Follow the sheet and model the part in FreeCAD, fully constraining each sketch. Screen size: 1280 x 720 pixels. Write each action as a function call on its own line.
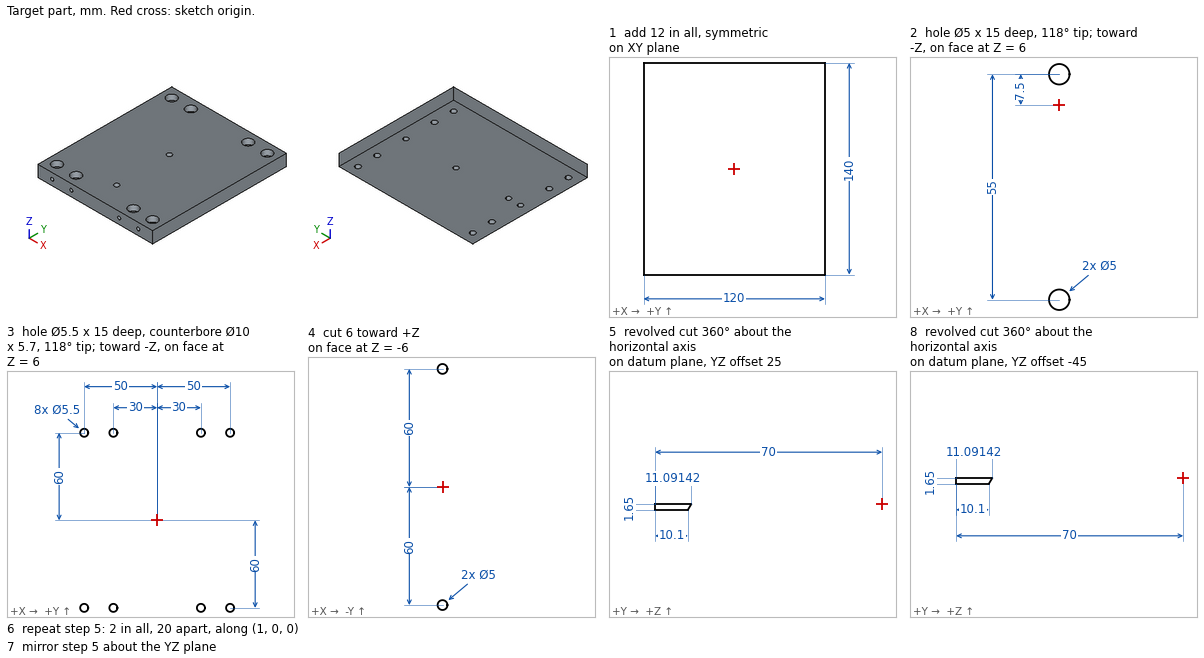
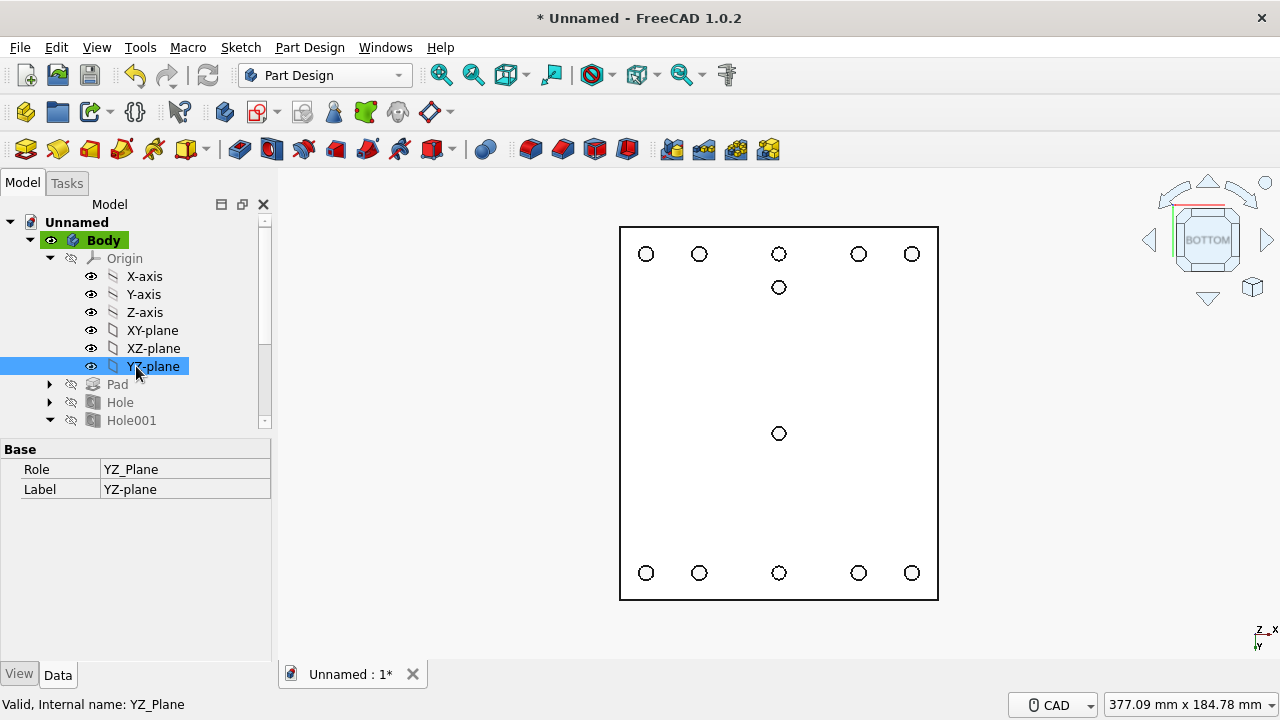
click(430, 112)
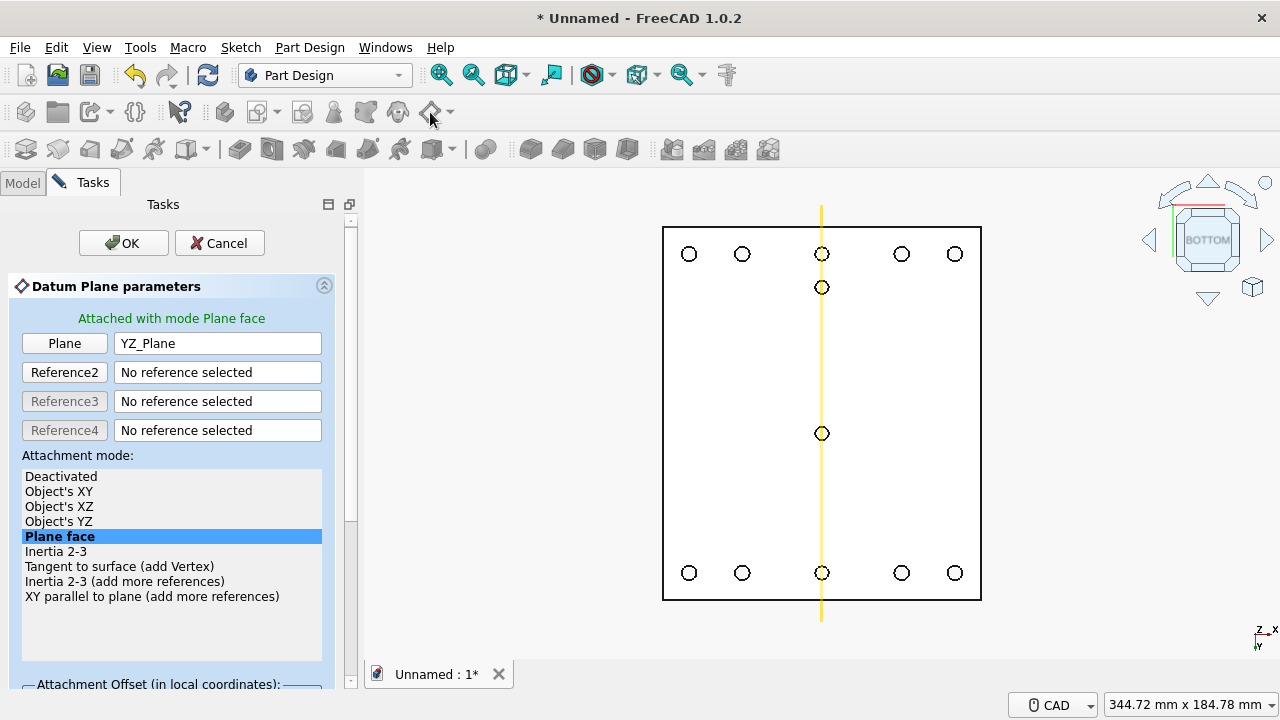
scroll(351, 451, down, 3)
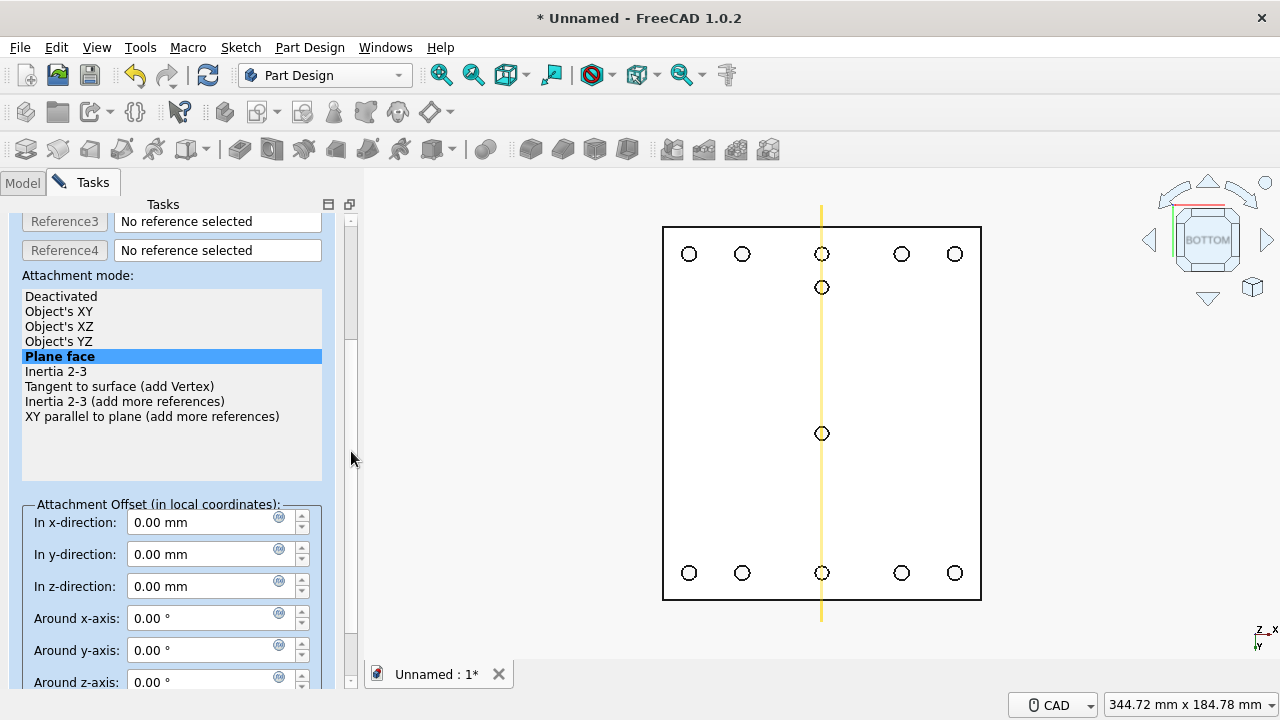
triple_click(210, 586)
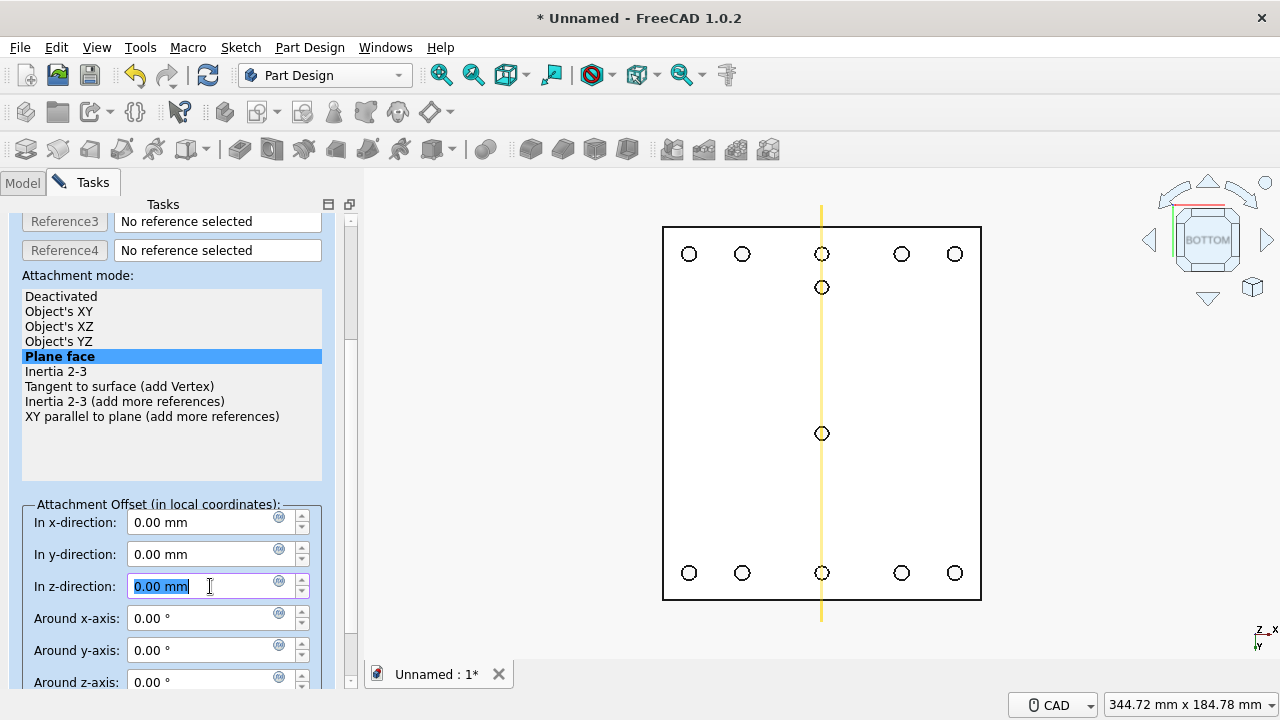
text(-45)
key(Tab)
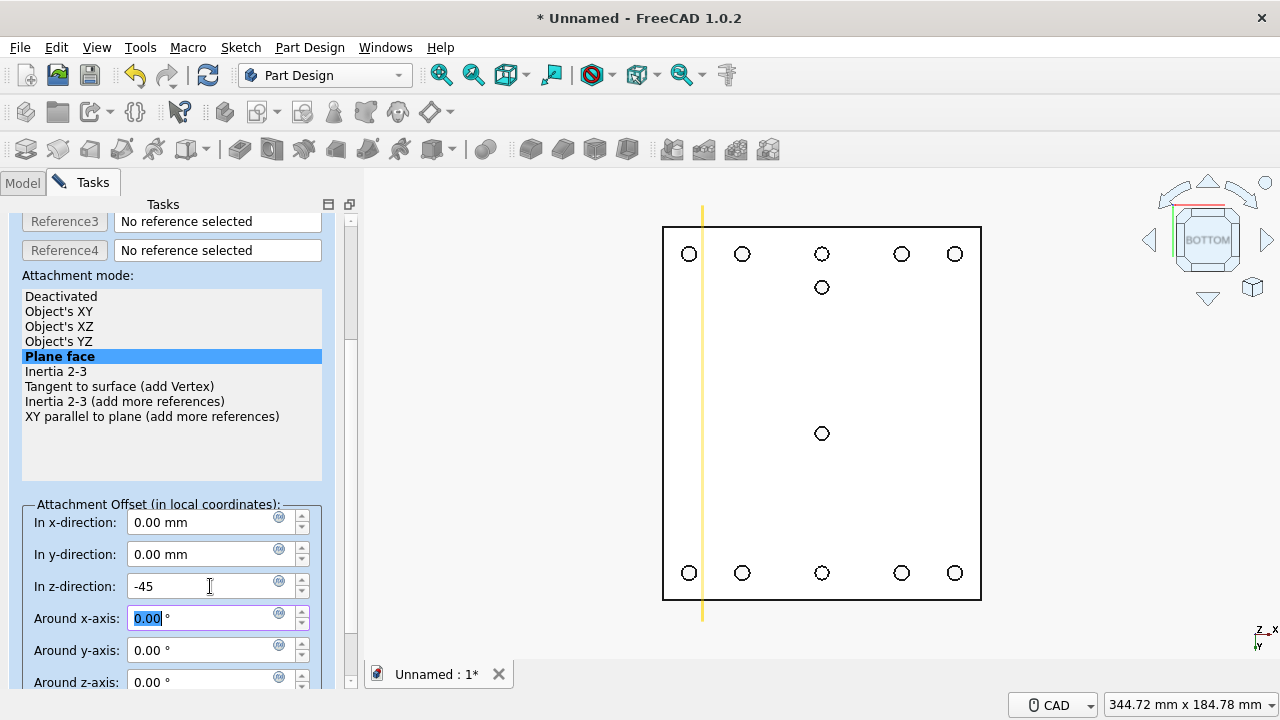
scroll(351, 451, up, 4)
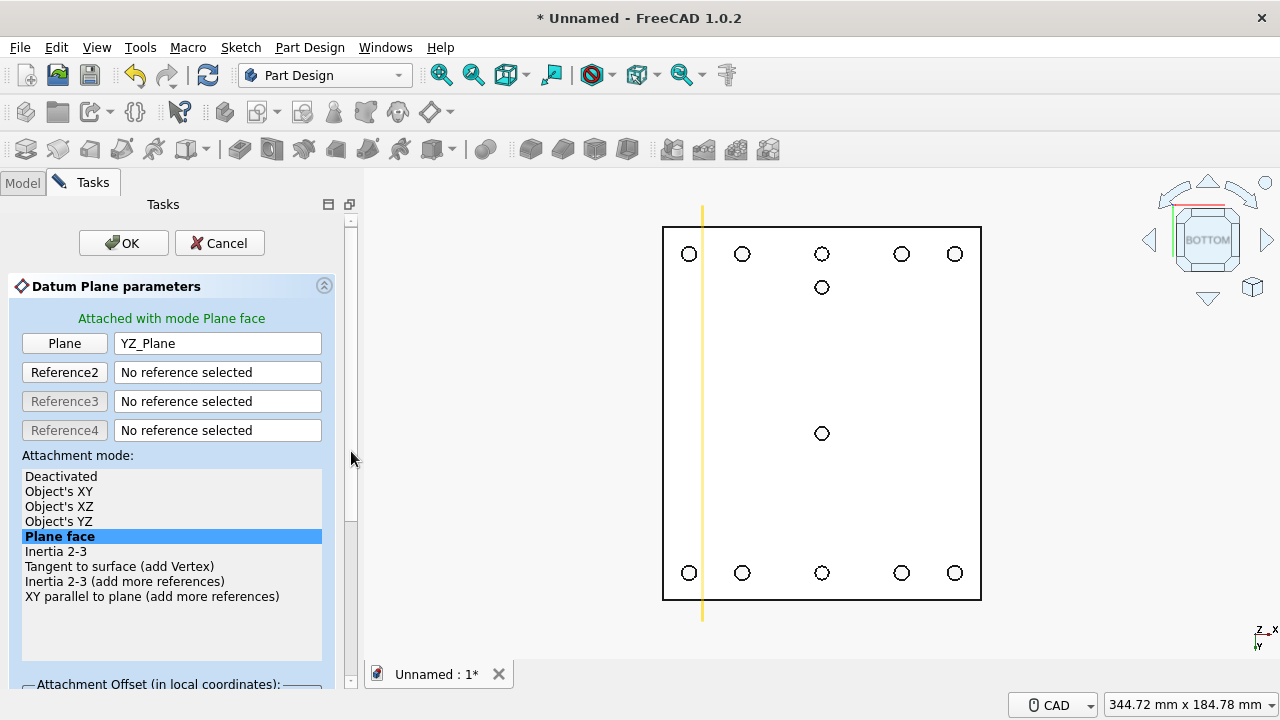
click(124, 243)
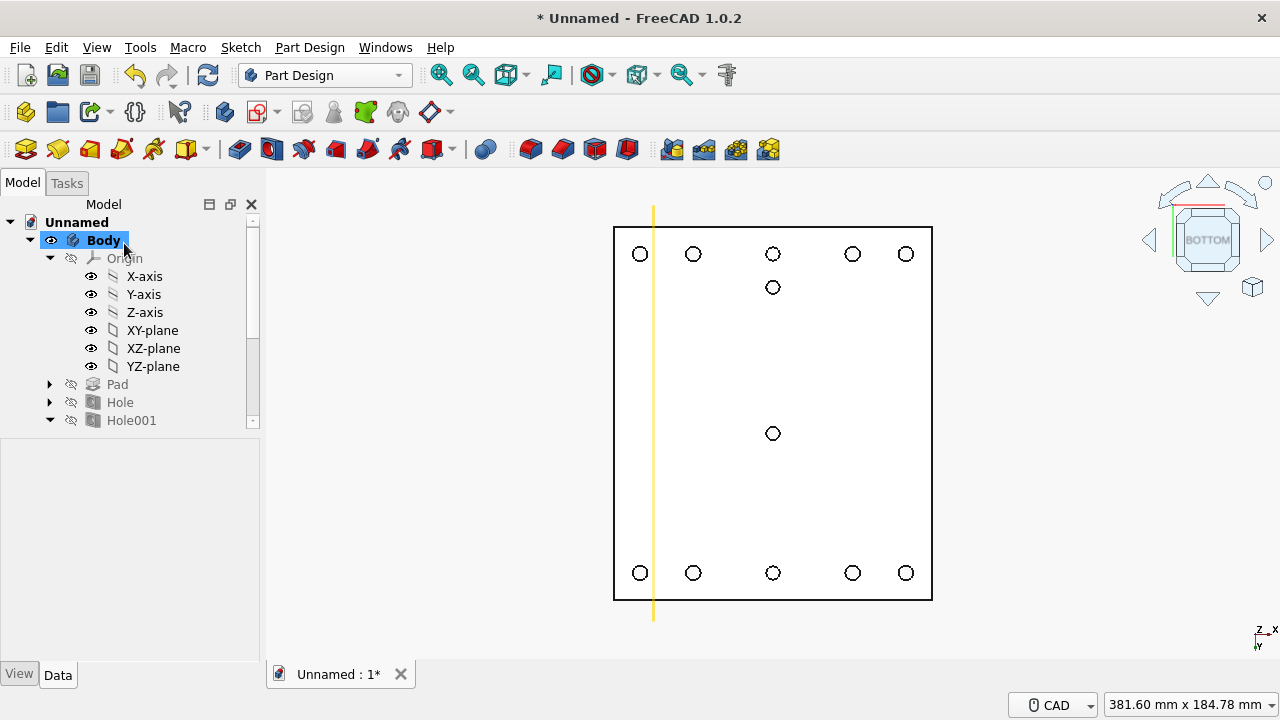
scroll(100, 326, down, 3)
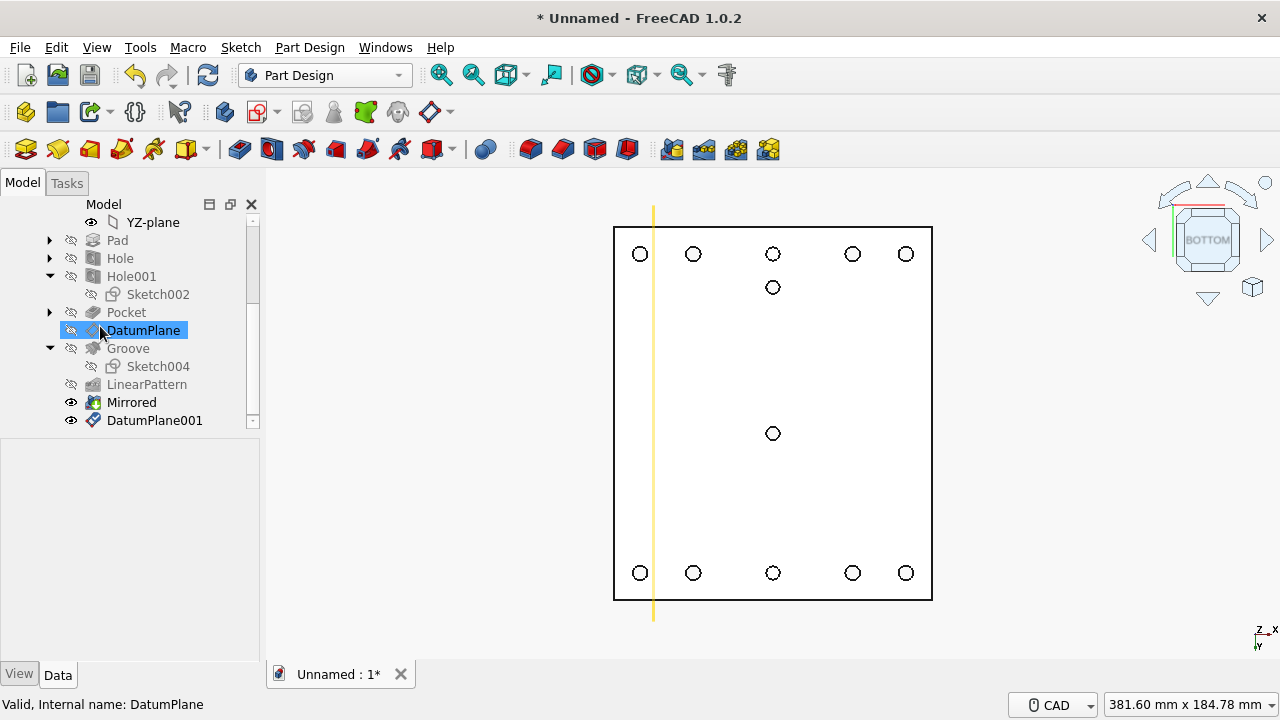
click(116, 420)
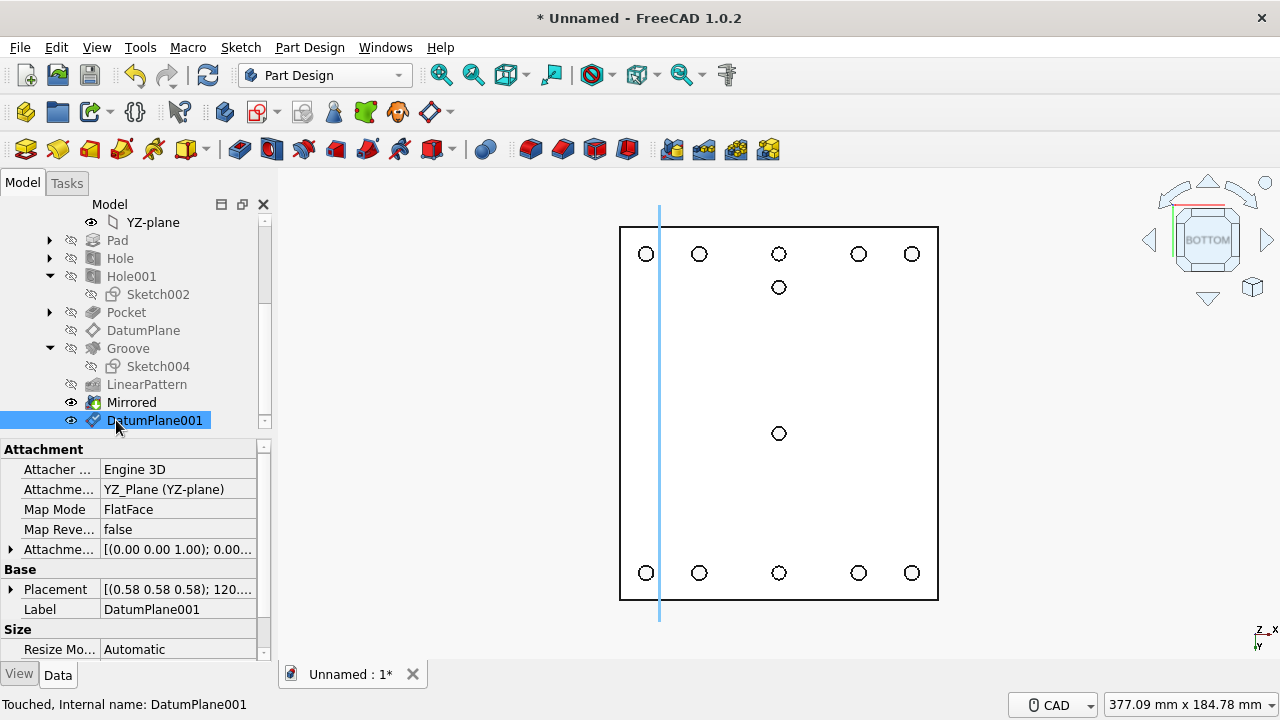
click(258, 112)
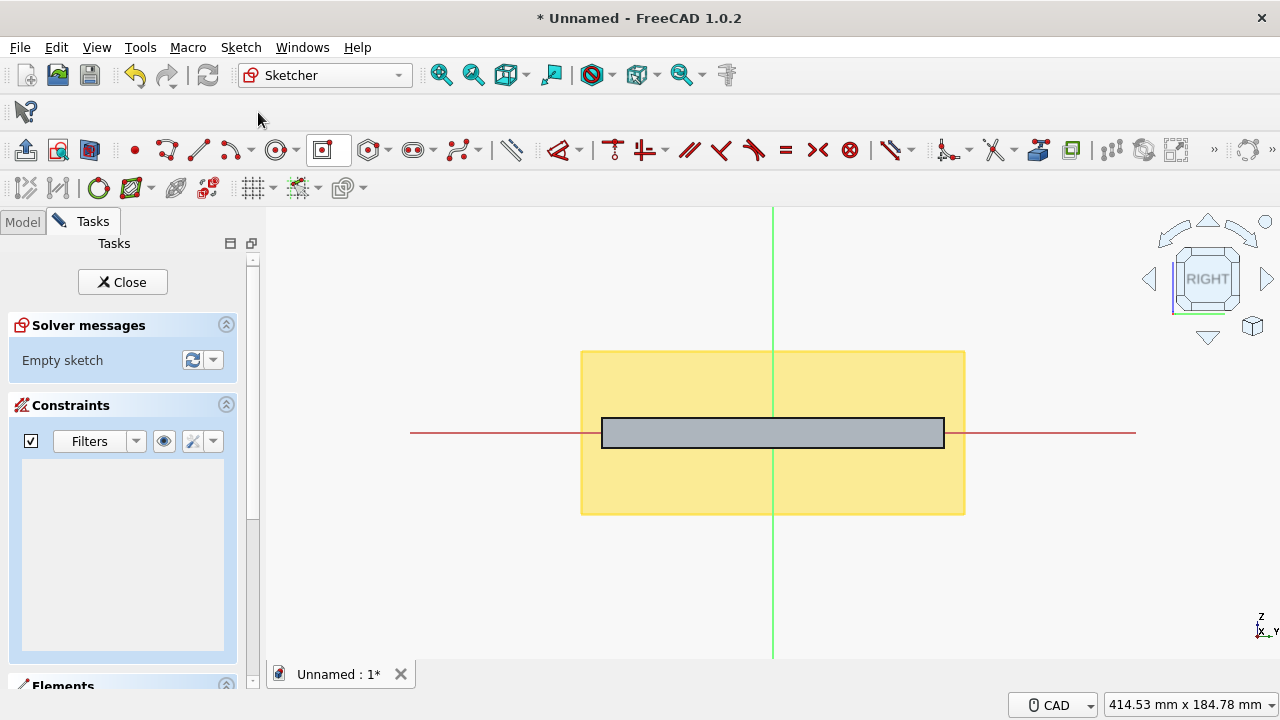
click(90, 150)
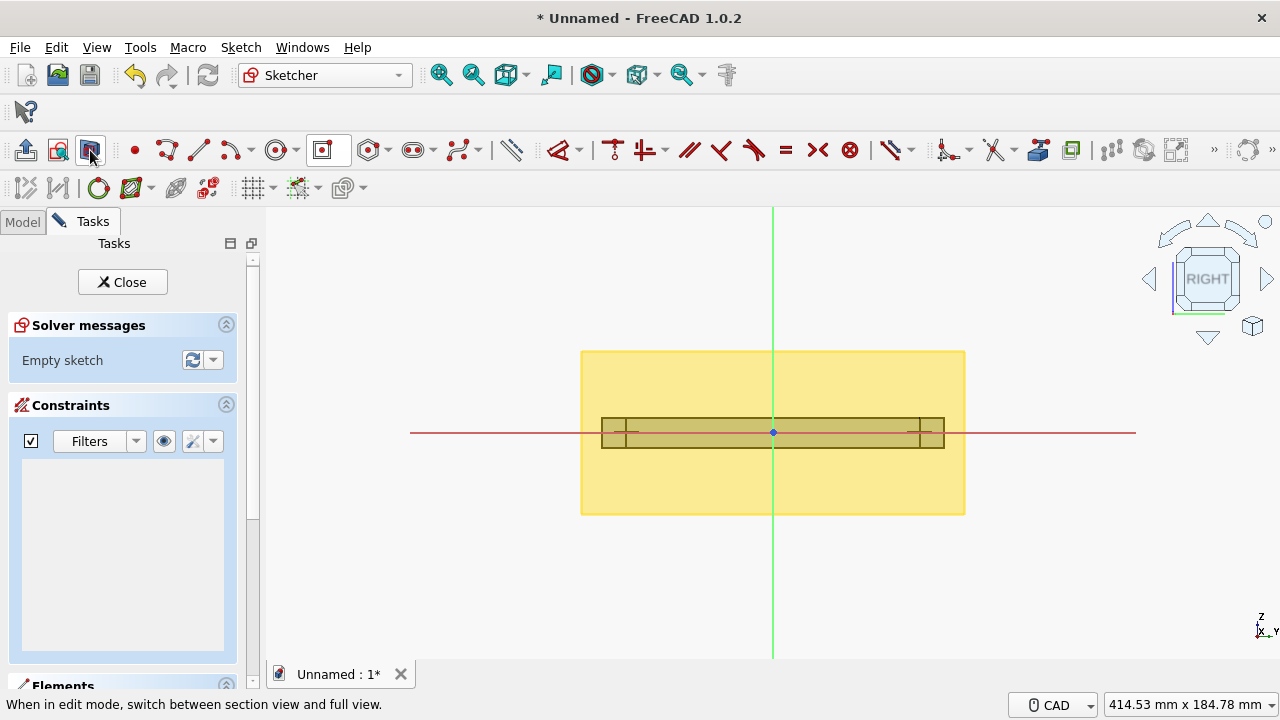
scroll(611, 435, up, 15)